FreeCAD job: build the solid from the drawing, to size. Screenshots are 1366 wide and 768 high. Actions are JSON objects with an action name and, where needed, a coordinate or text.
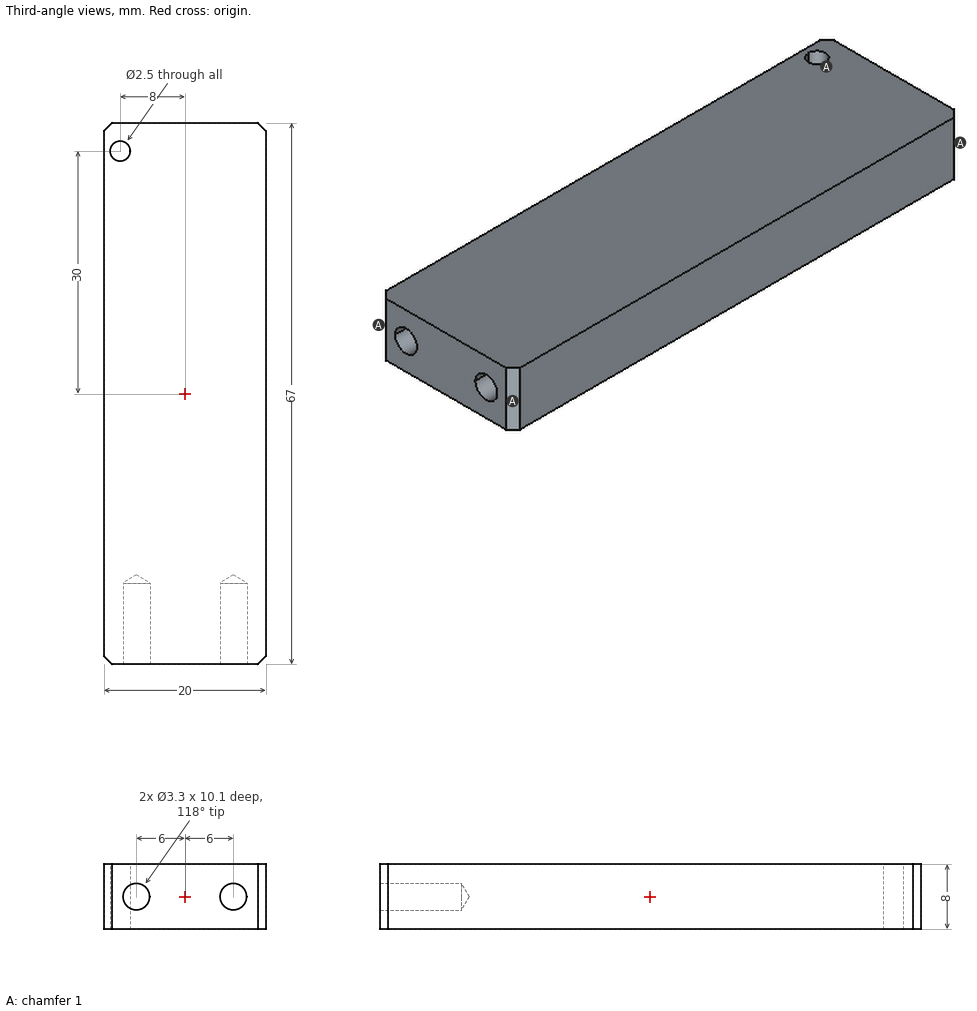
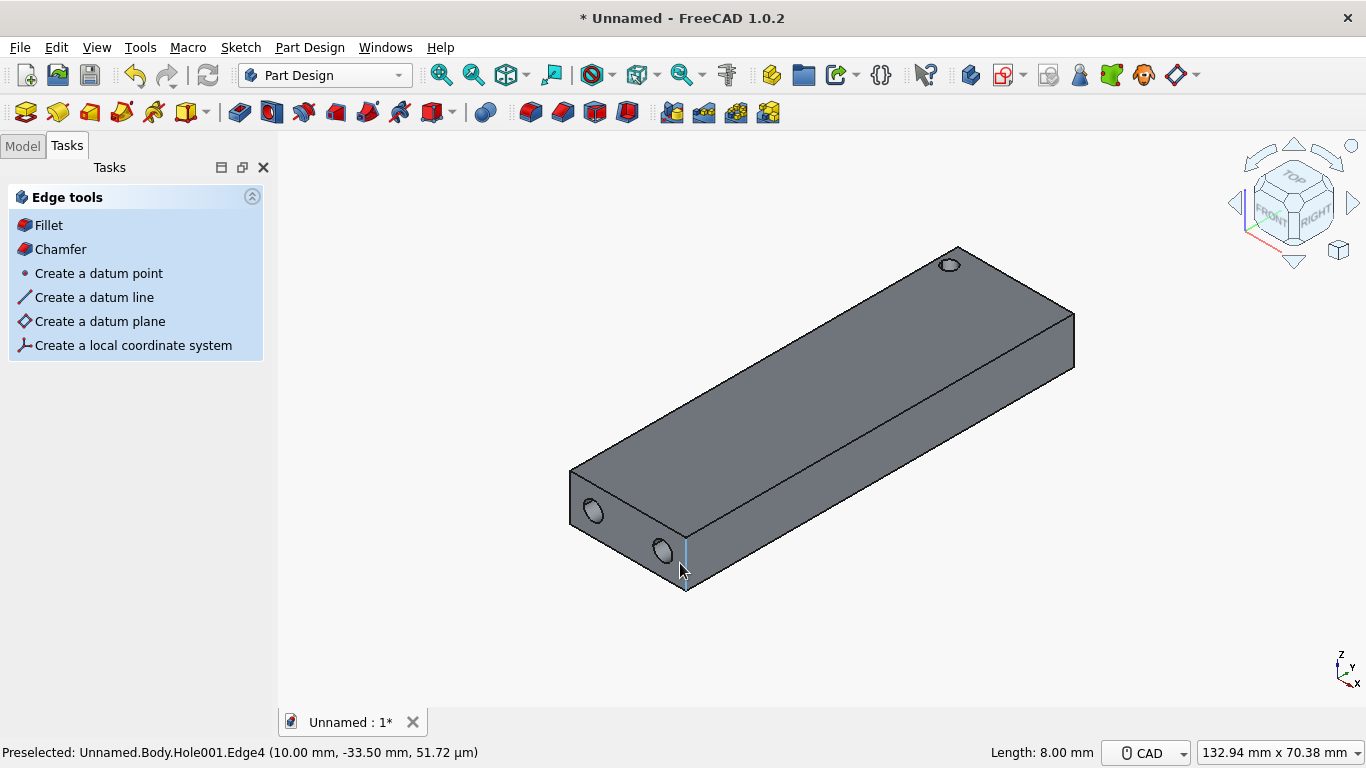
{"action": "key", "text": "2"}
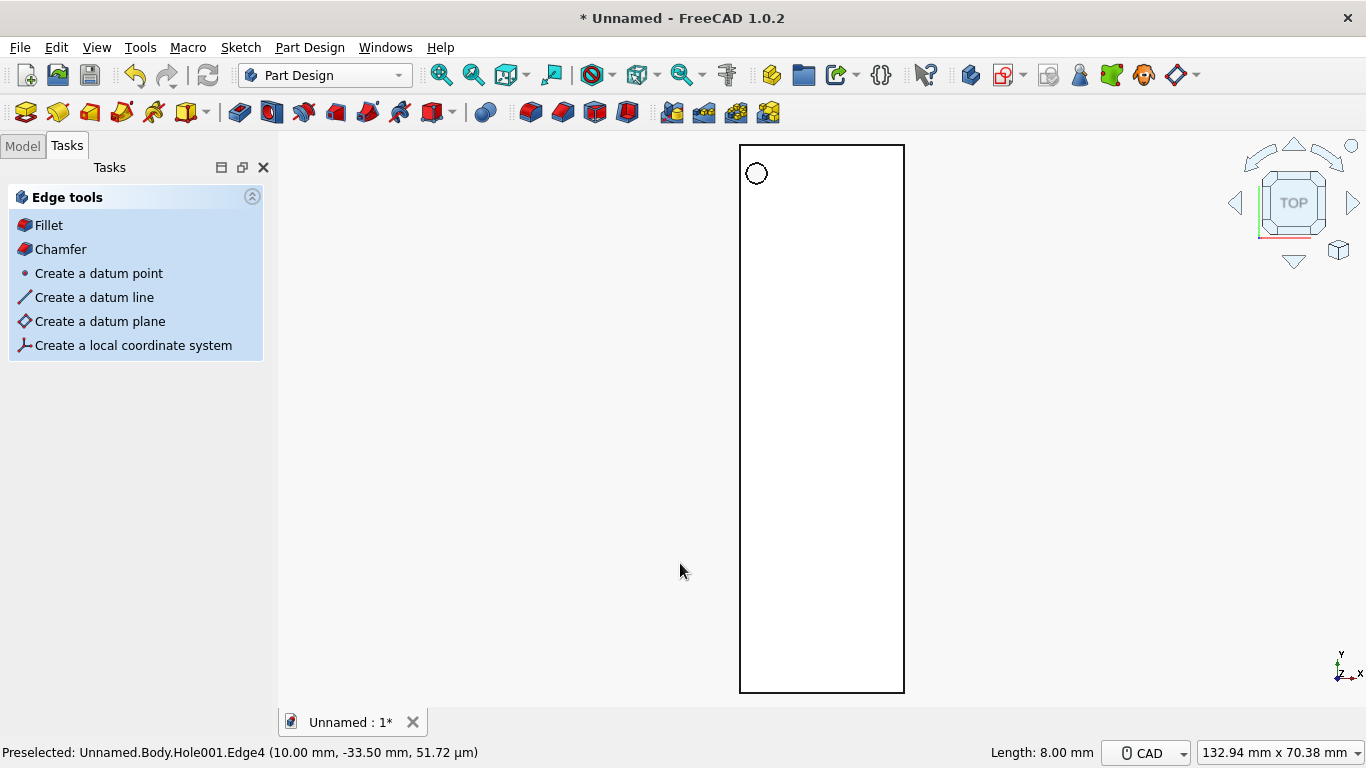
{"action": "key", "text": "0"}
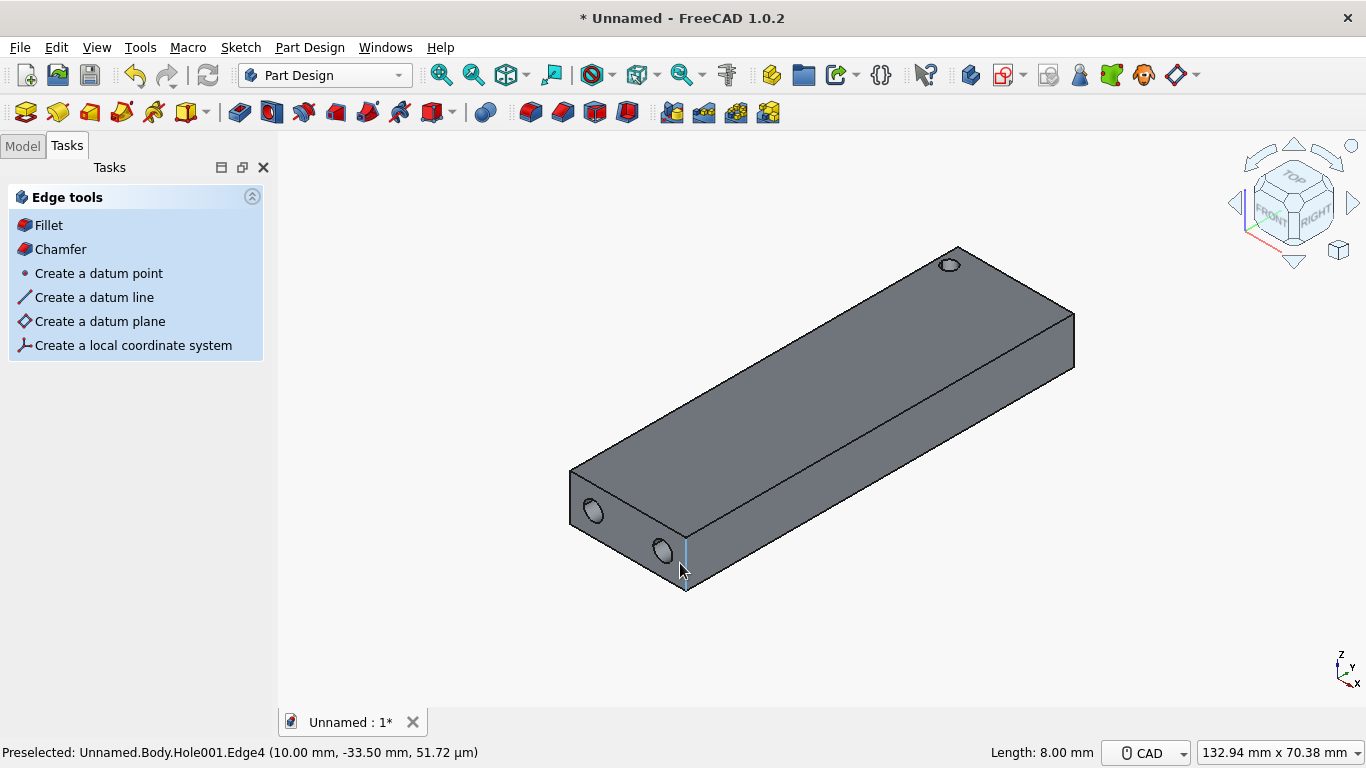
{"action": "key", "text": "1"}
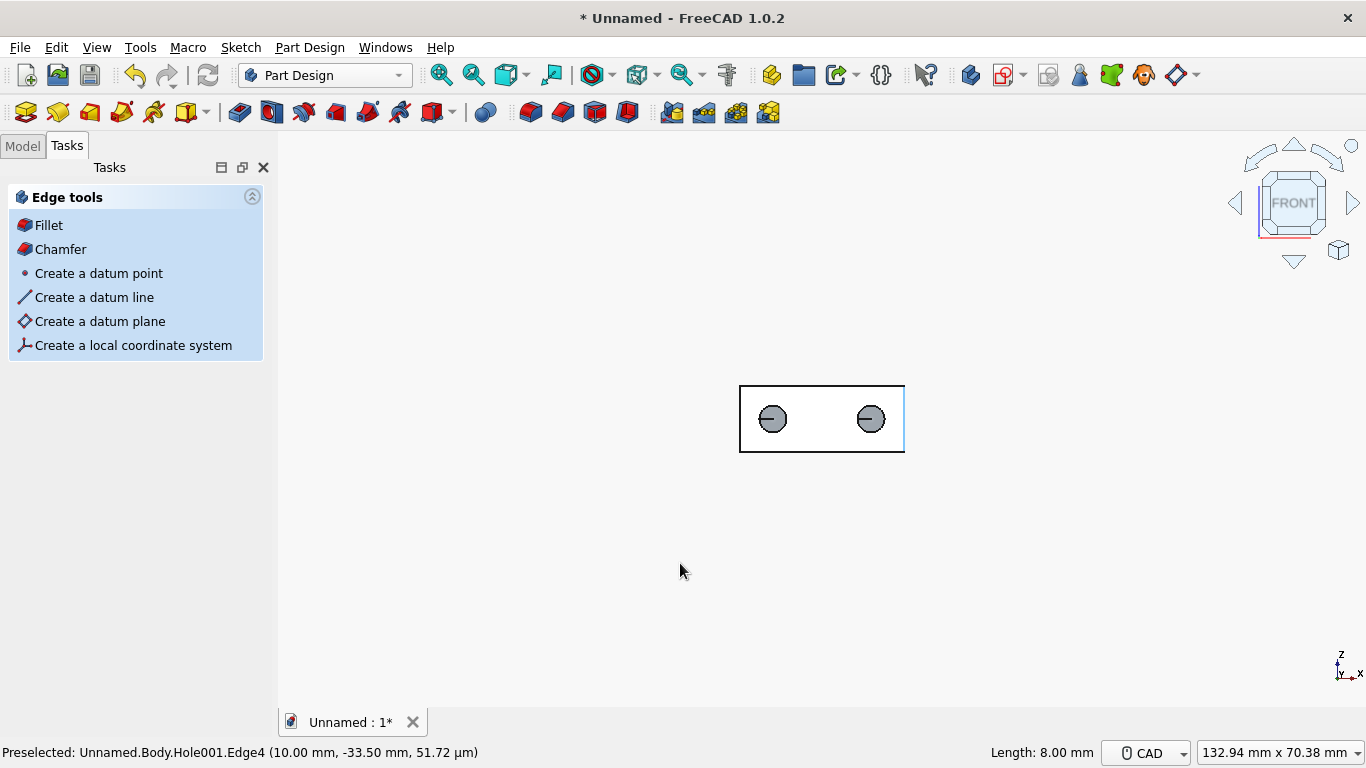
{"action": "key", "text": "v f"}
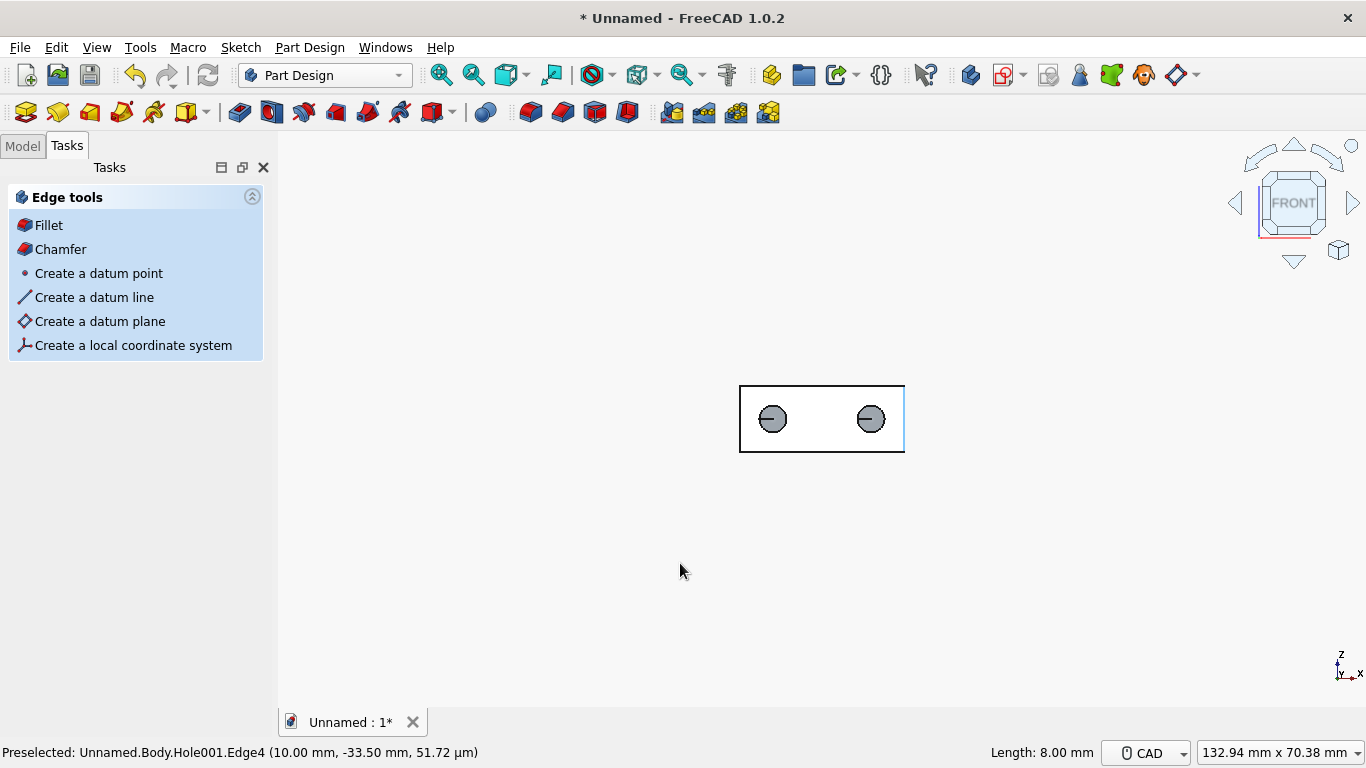
{"action": "left_click", "coordinate": [740, 418], "text": "ctrl"}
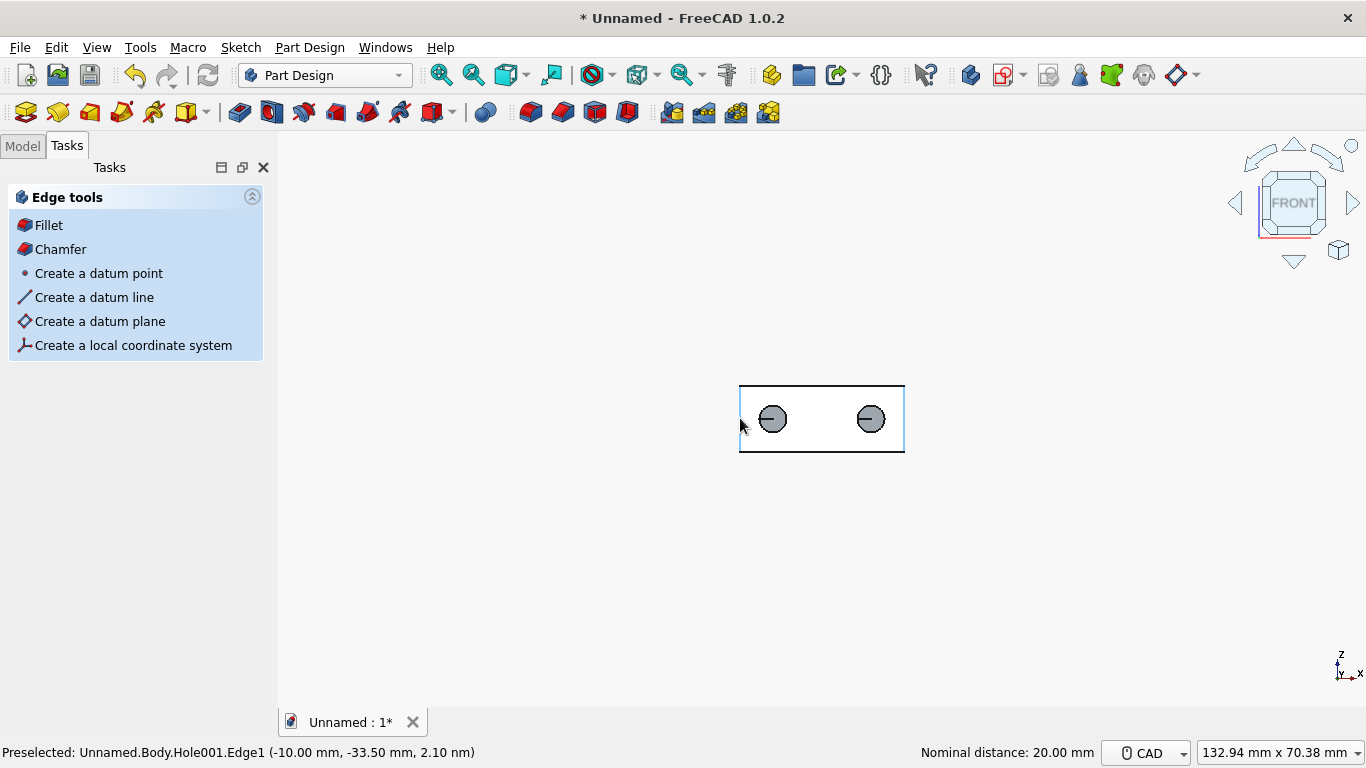
{"action": "key", "text": "3"}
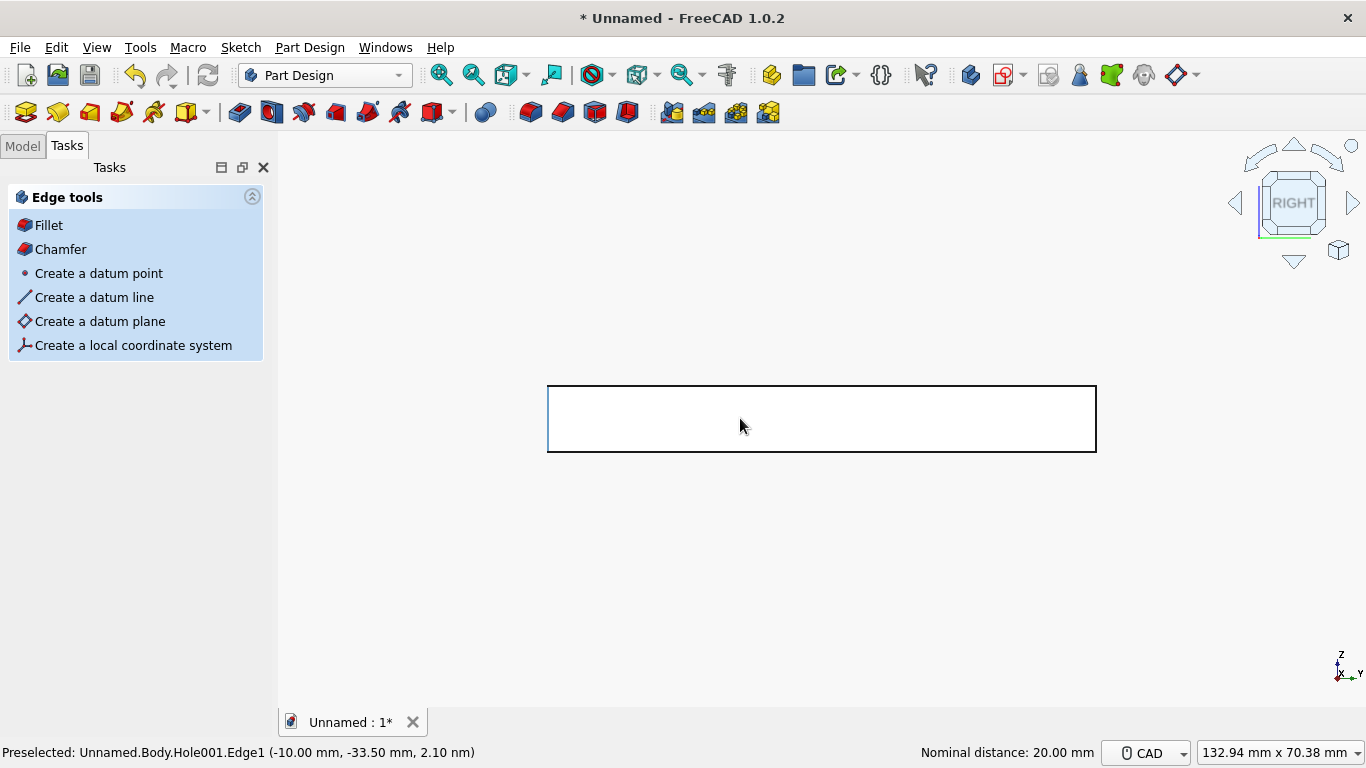
{"action": "left_click", "coordinate": [1096, 418], "text": "ctrl"}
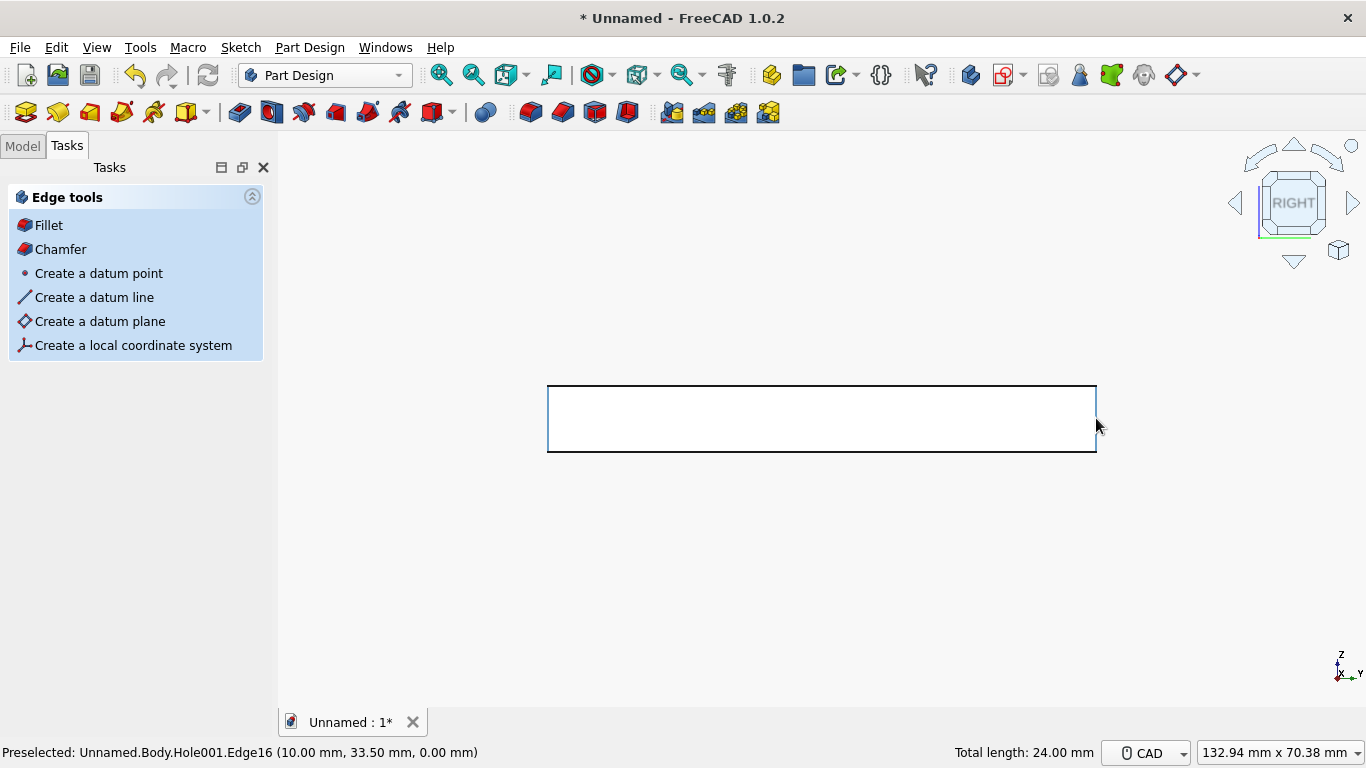
{"action": "key", "text": "5"}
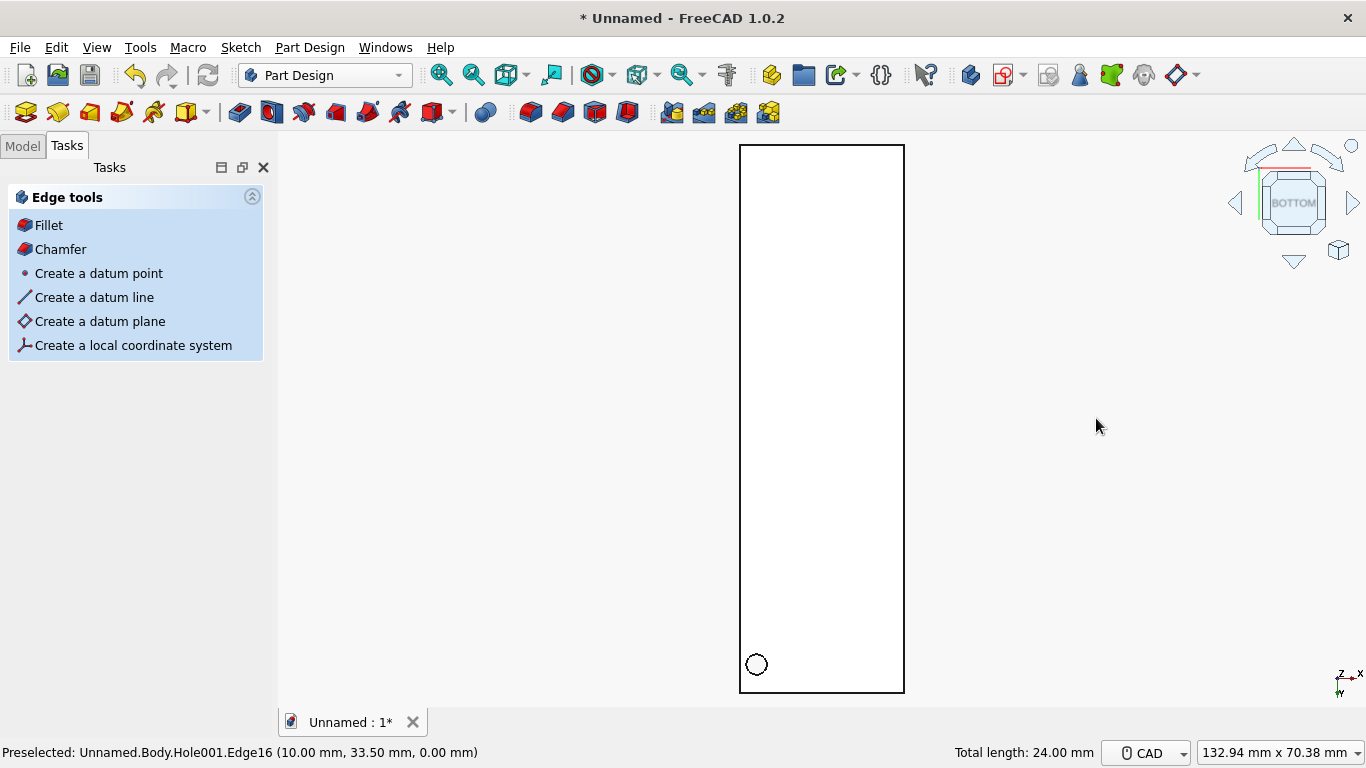
{"action": "key", "text": "4"}